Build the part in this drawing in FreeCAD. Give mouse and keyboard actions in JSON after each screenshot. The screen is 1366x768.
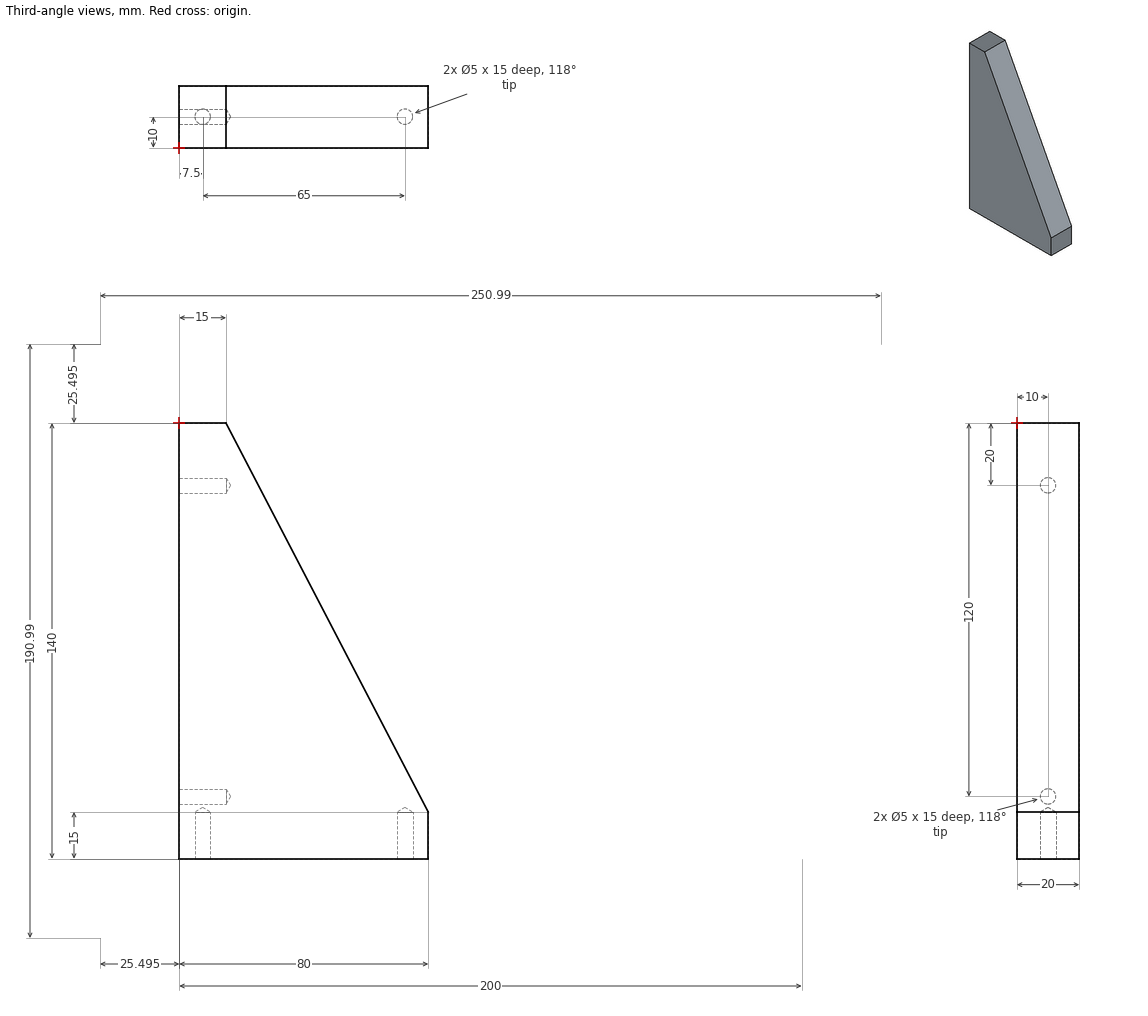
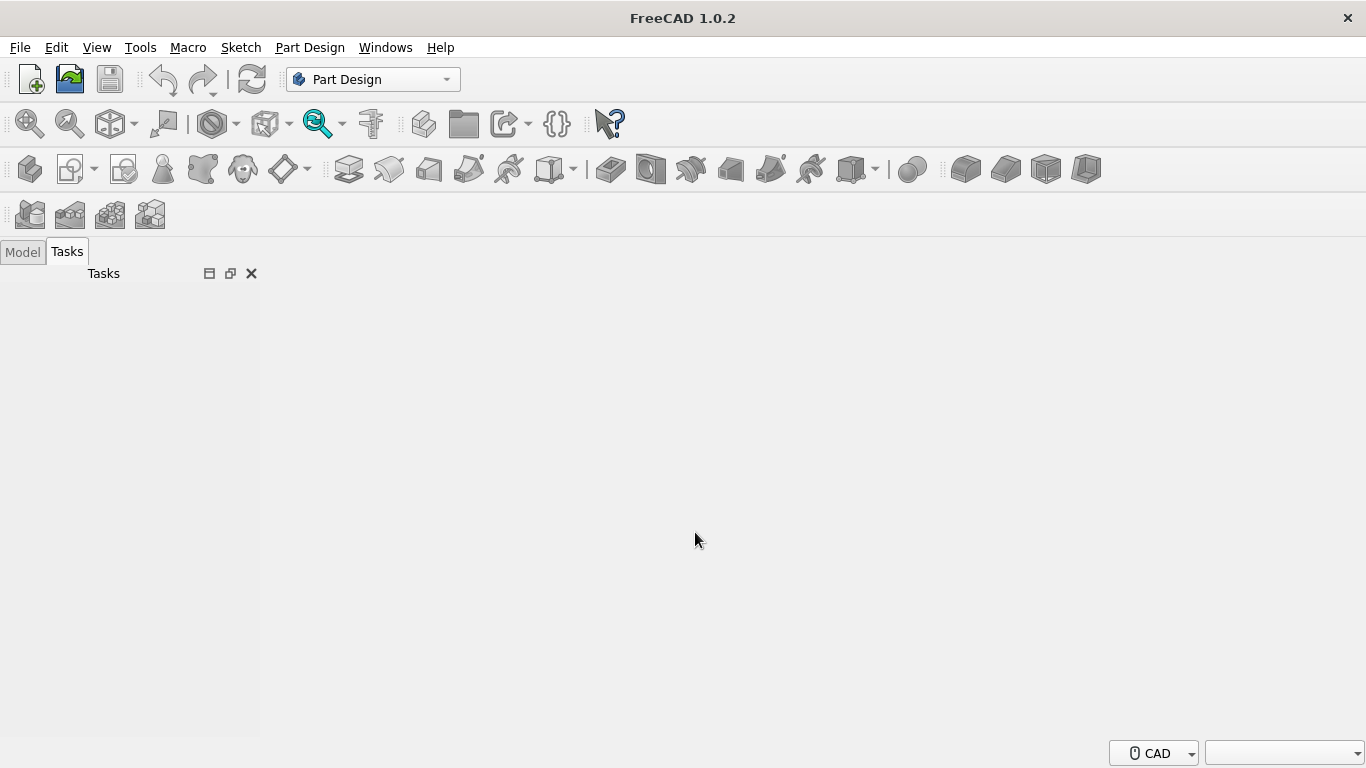
{"action": "key", "text": "ctrl+n"}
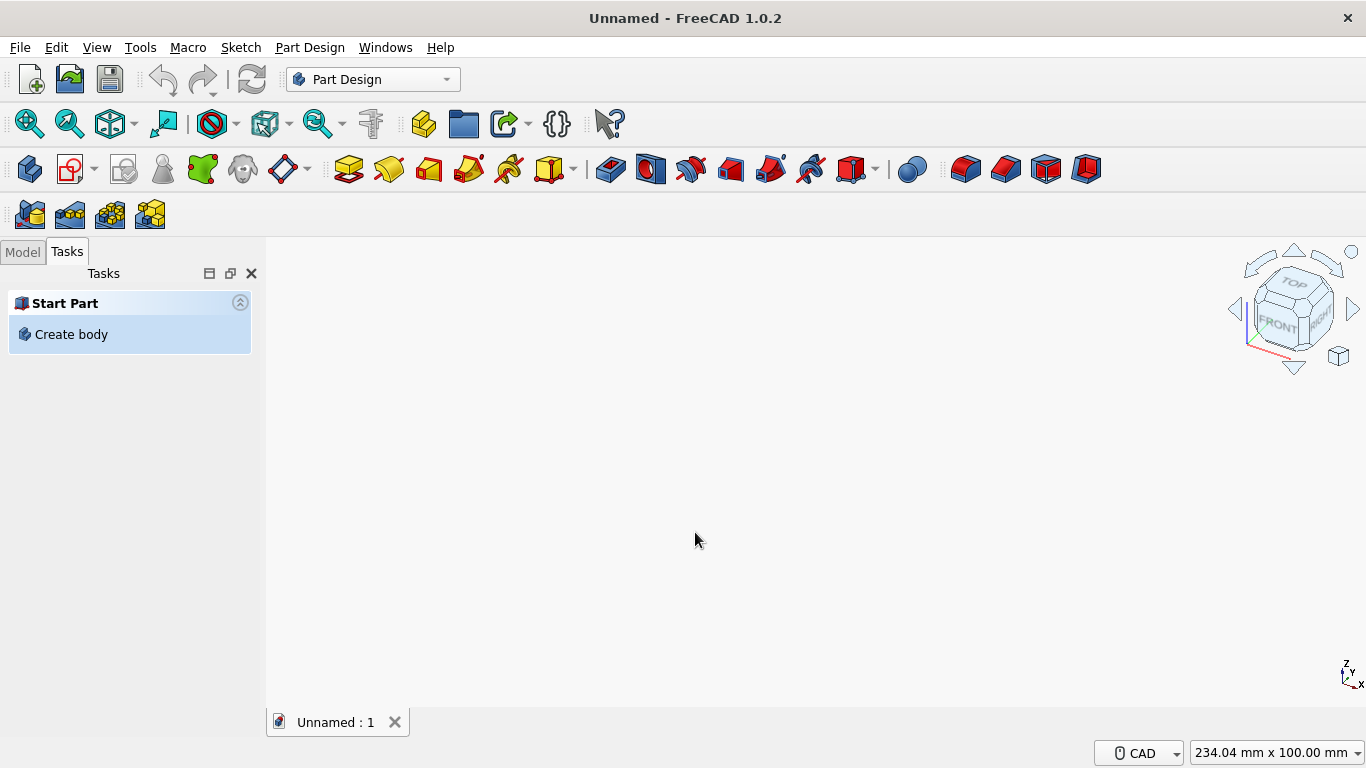
{"action": "left_click", "coordinate": [70, 170]}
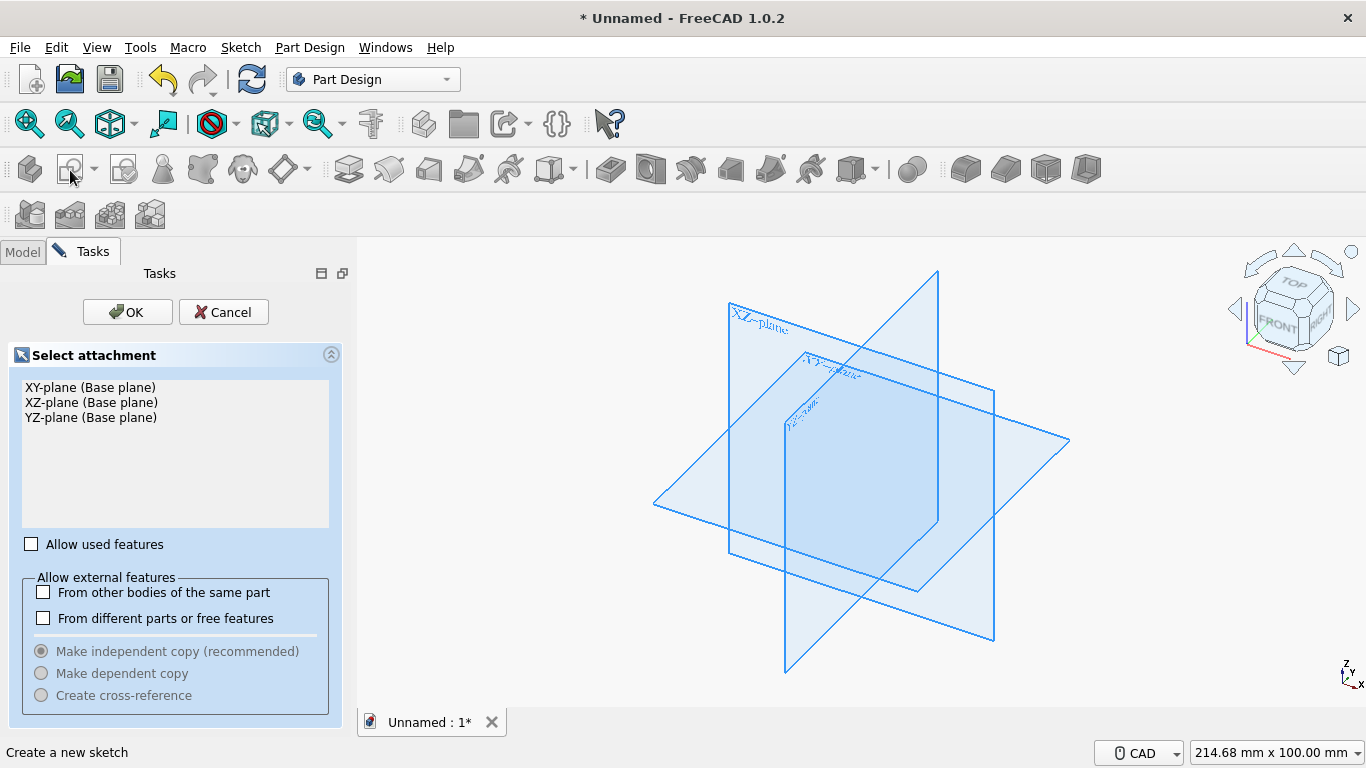
{"action": "left_click", "coordinate": [82, 402]}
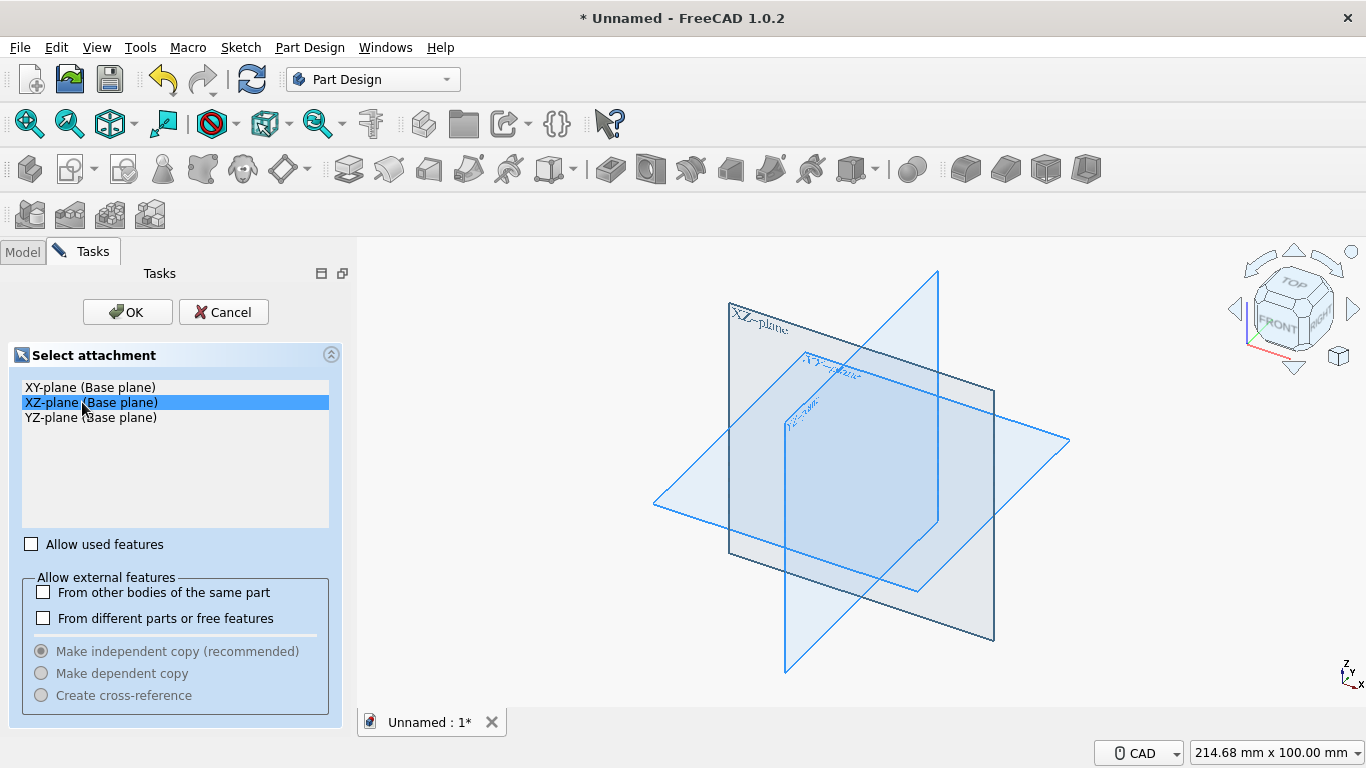
{"action": "left_click", "coordinate": [128, 312]}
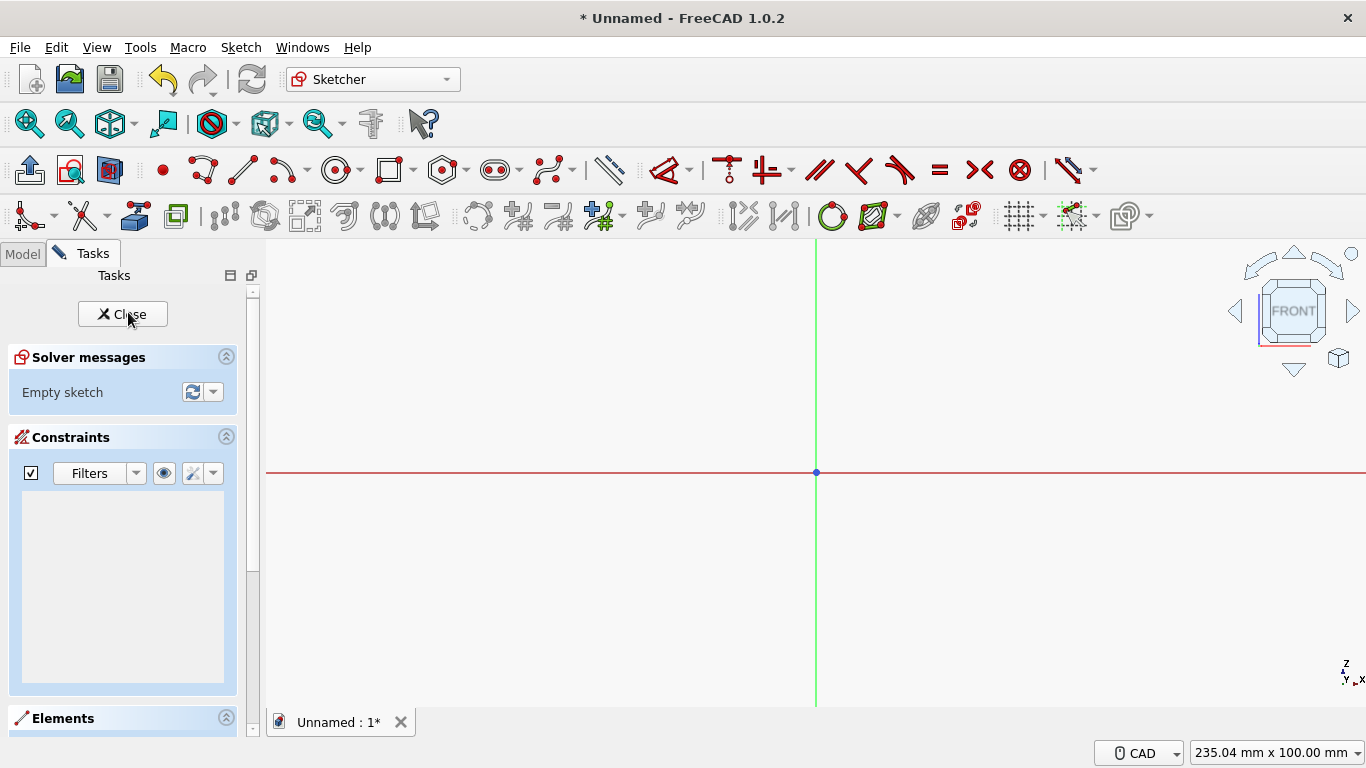
{"action": "scroll", "coordinate": [310, 267], "scroll_direction": "down", "scroll_amount": 4}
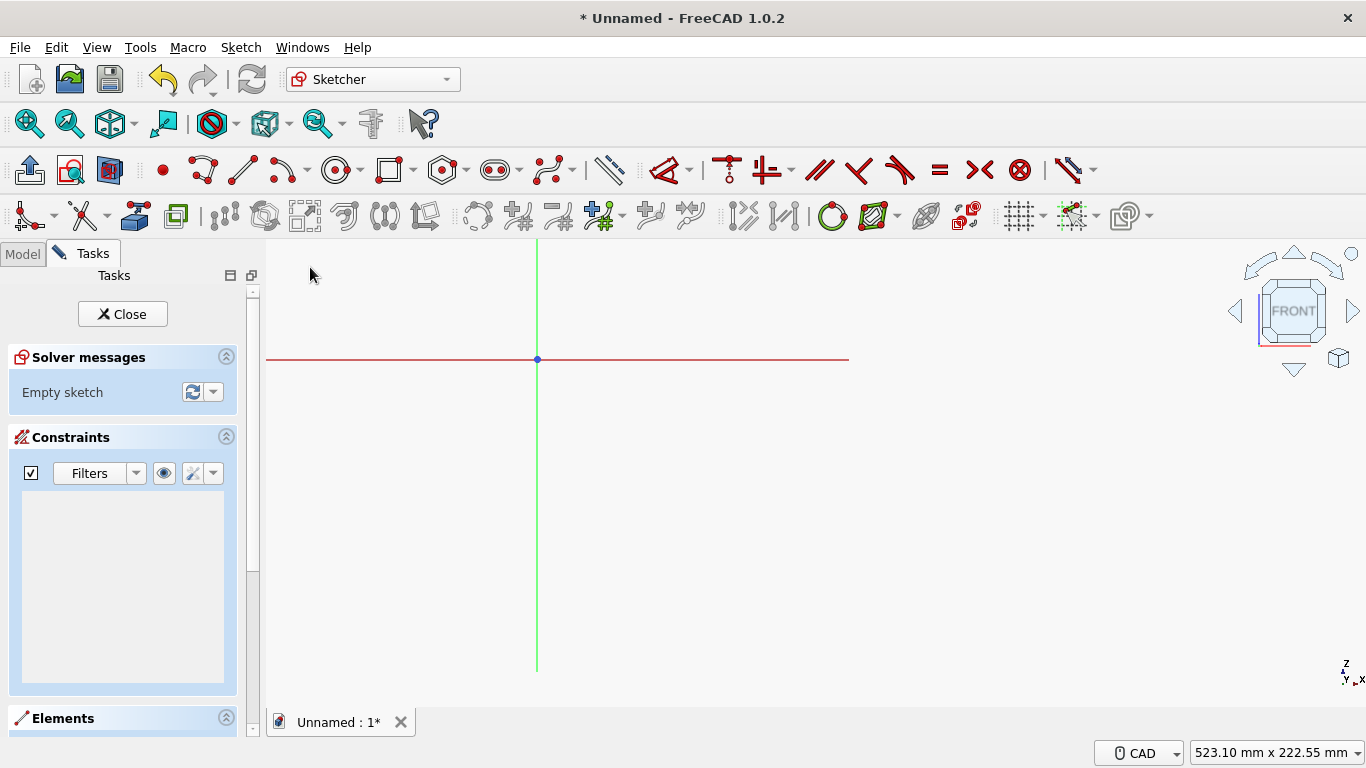
{"action": "key", "text": "g r"}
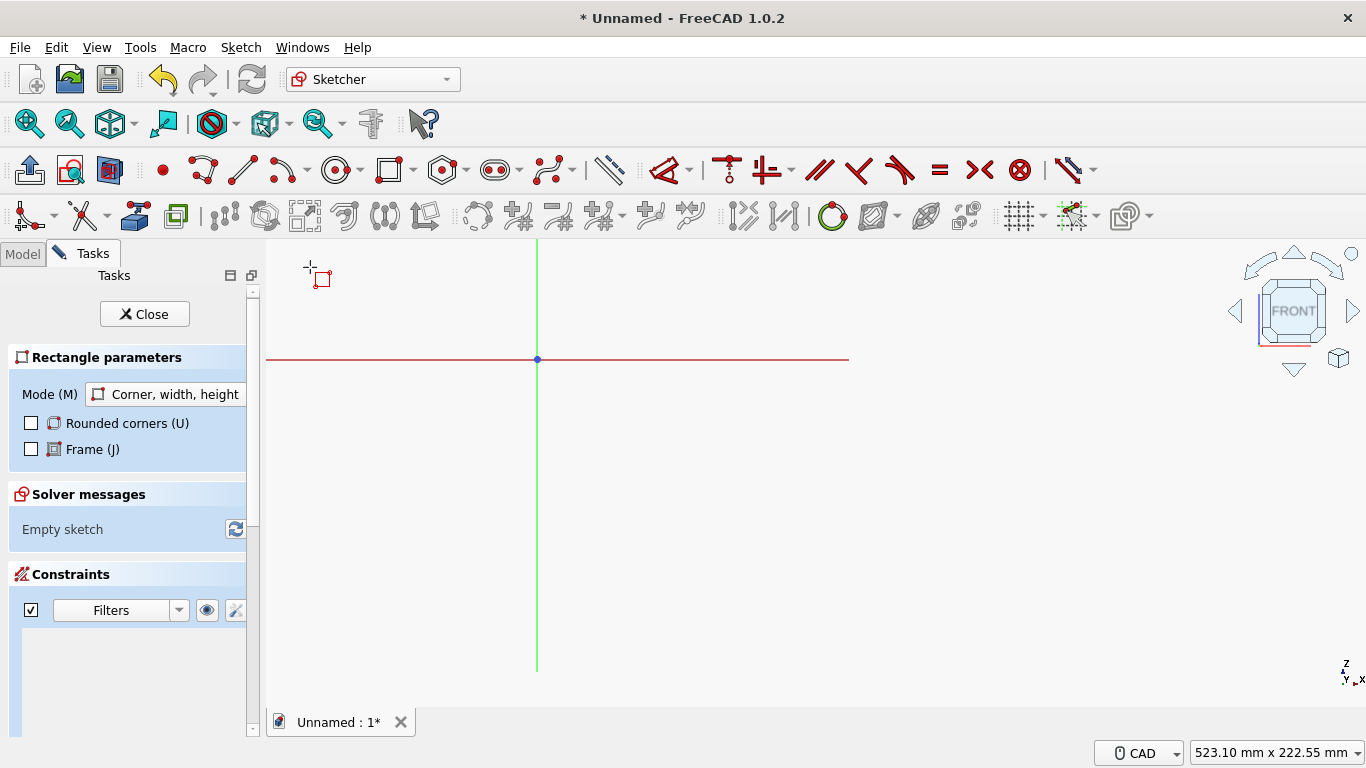
{"action": "left_click", "coordinate": [537, 360]}
{"action": "left_click", "coordinate": [958, 654]}
{"action": "key", "text": "Escape"}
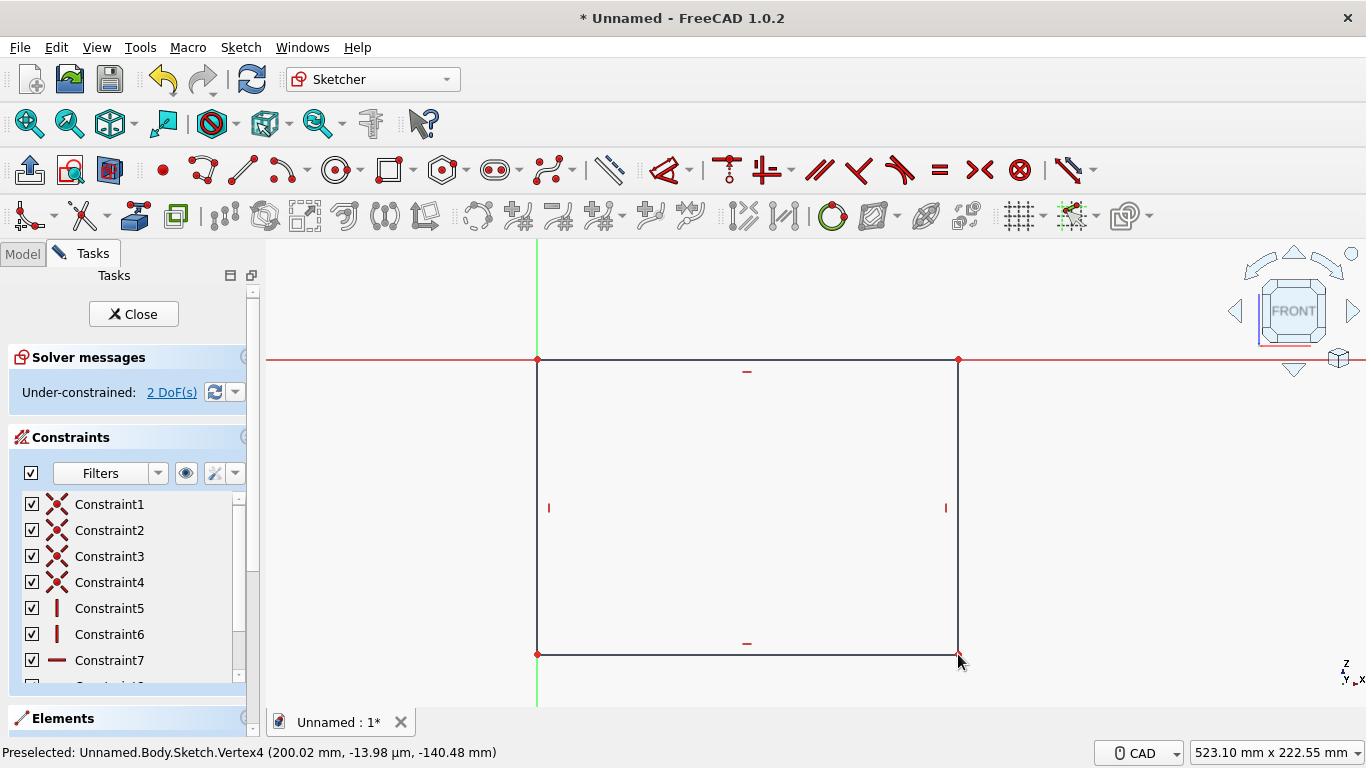
{"action": "key", "text": "d"}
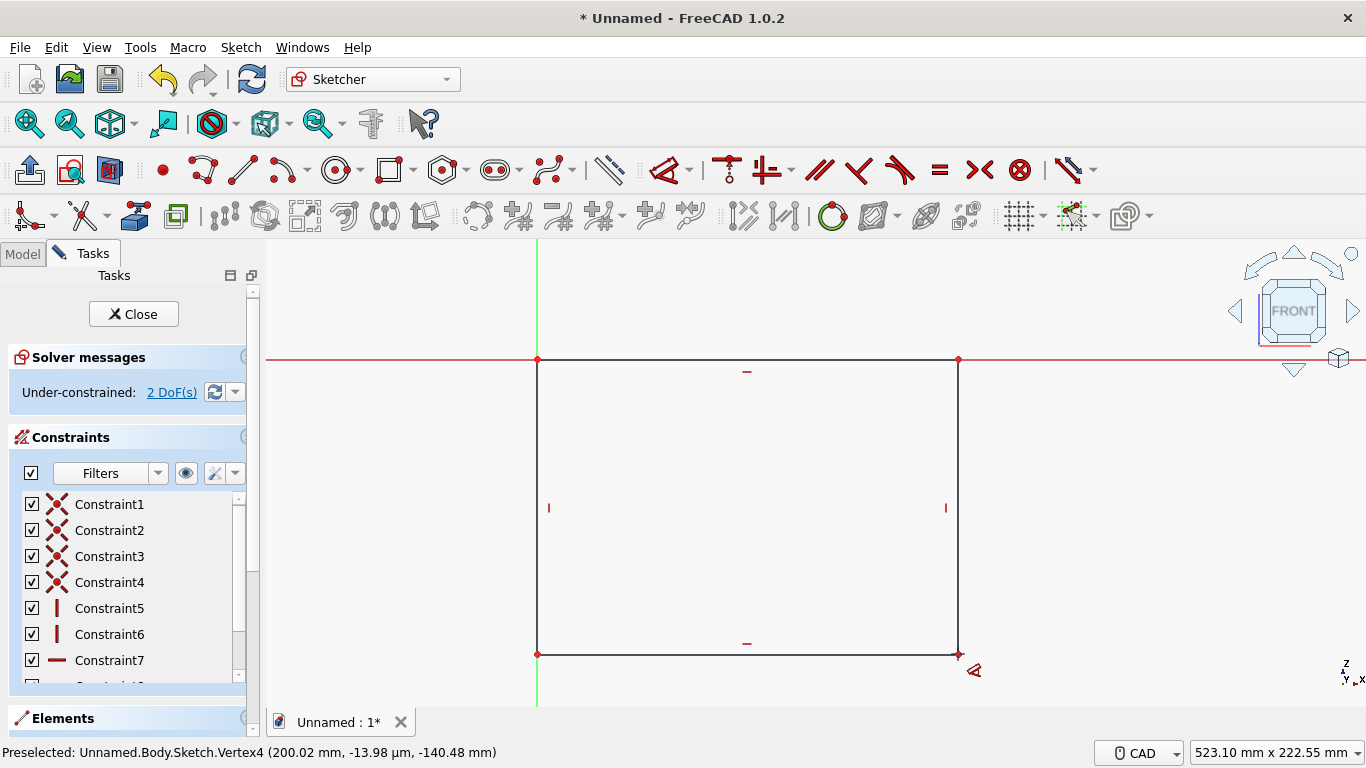
{"action": "left_click", "coordinate": [537, 448]}
{"action": "left_click", "coordinate": [503, 507]}